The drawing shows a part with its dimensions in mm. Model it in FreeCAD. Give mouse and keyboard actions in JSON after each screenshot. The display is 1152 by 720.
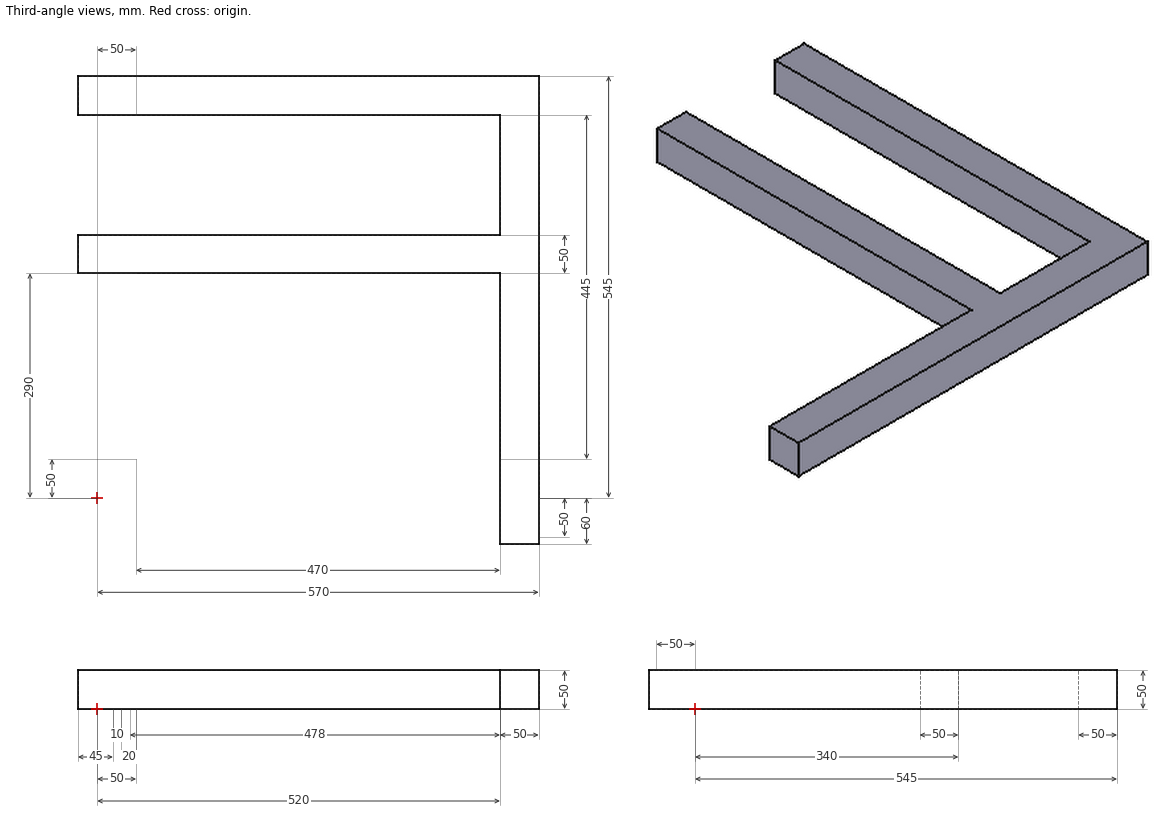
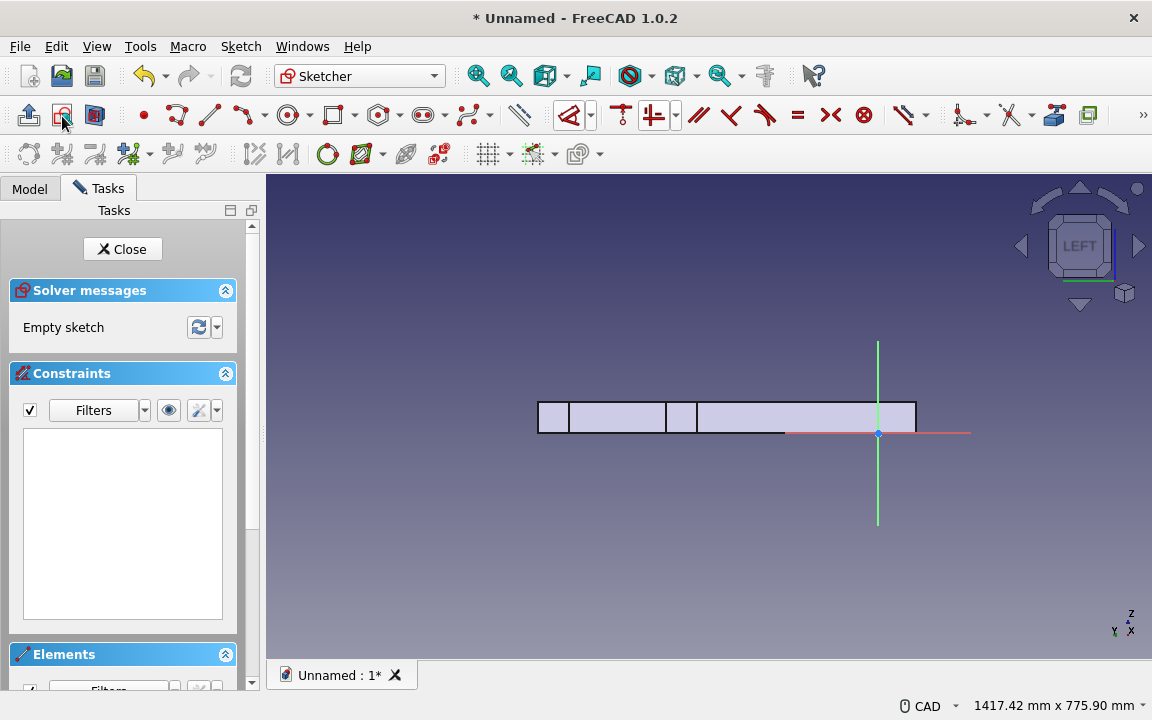
{"action": "scroll", "coordinate": [845, 420], "scroll_direction": "up", "scroll_amount": 2}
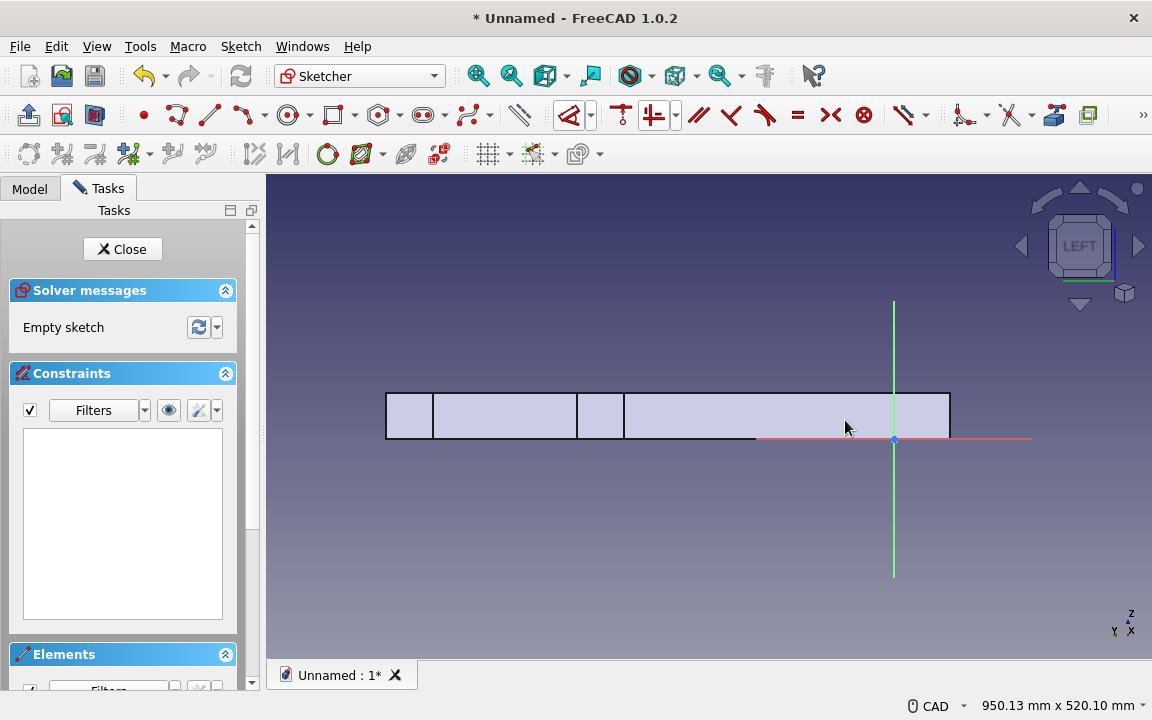
{"action": "key", "text": "g r"}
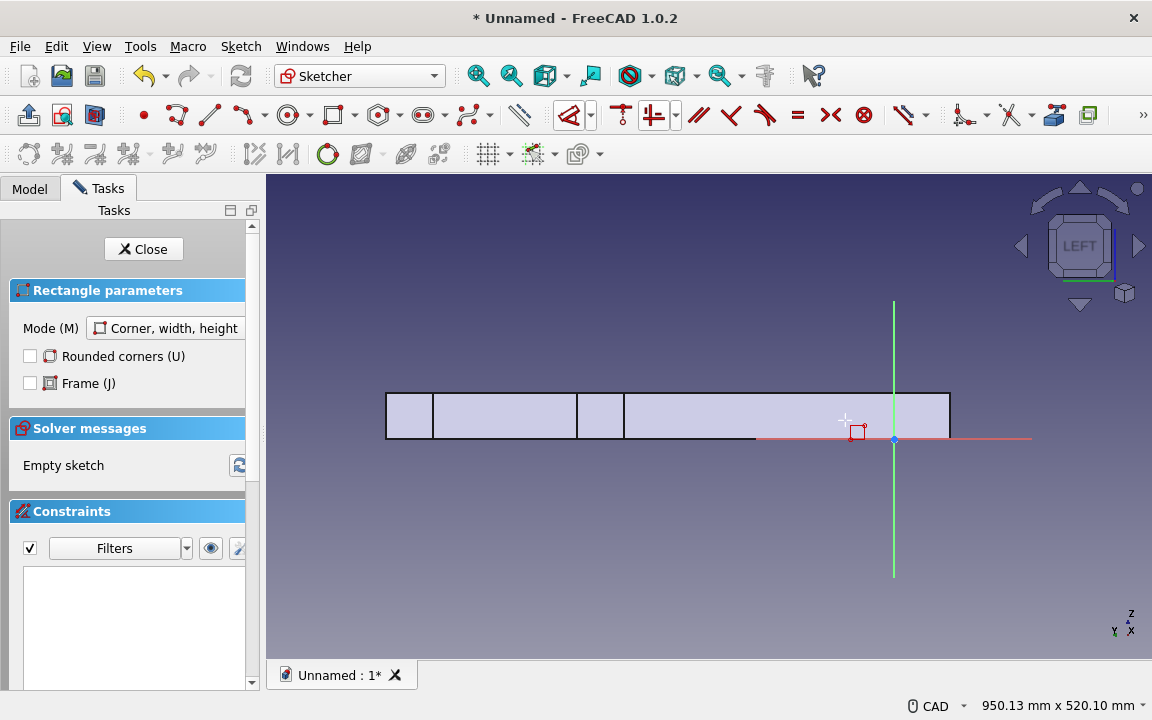
{"action": "left_click", "coordinate": [386, 393]}
{"action": "left_click", "coordinate": [433, 439]}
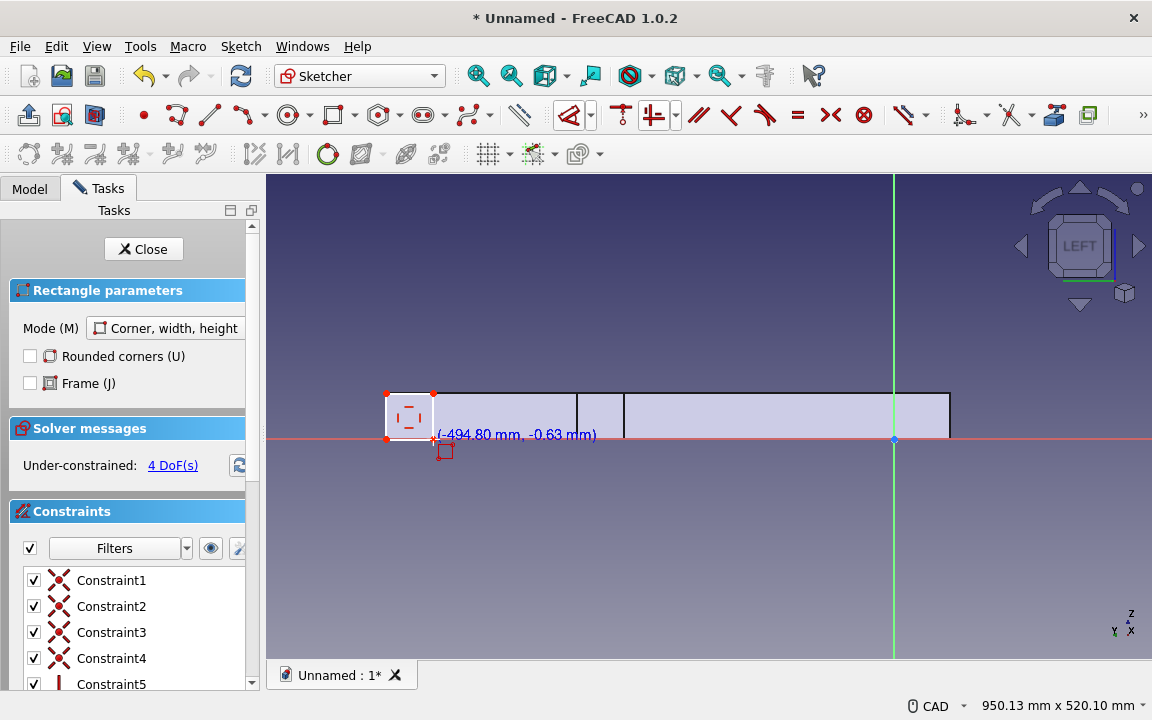
{"action": "left_click", "coordinate": [577, 393]}
{"action": "left_click", "coordinate": [624, 439]}
{"action": "key", "text": "Escape"}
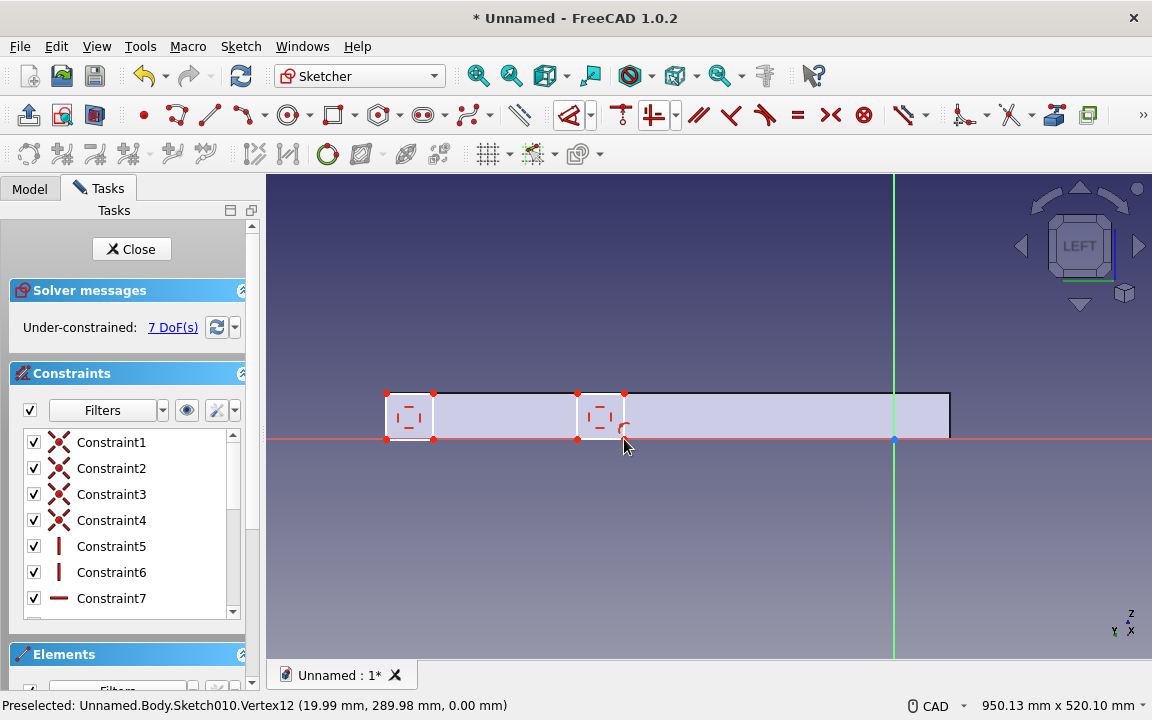
{"action": "left_click", "coordinate": [386, 440]}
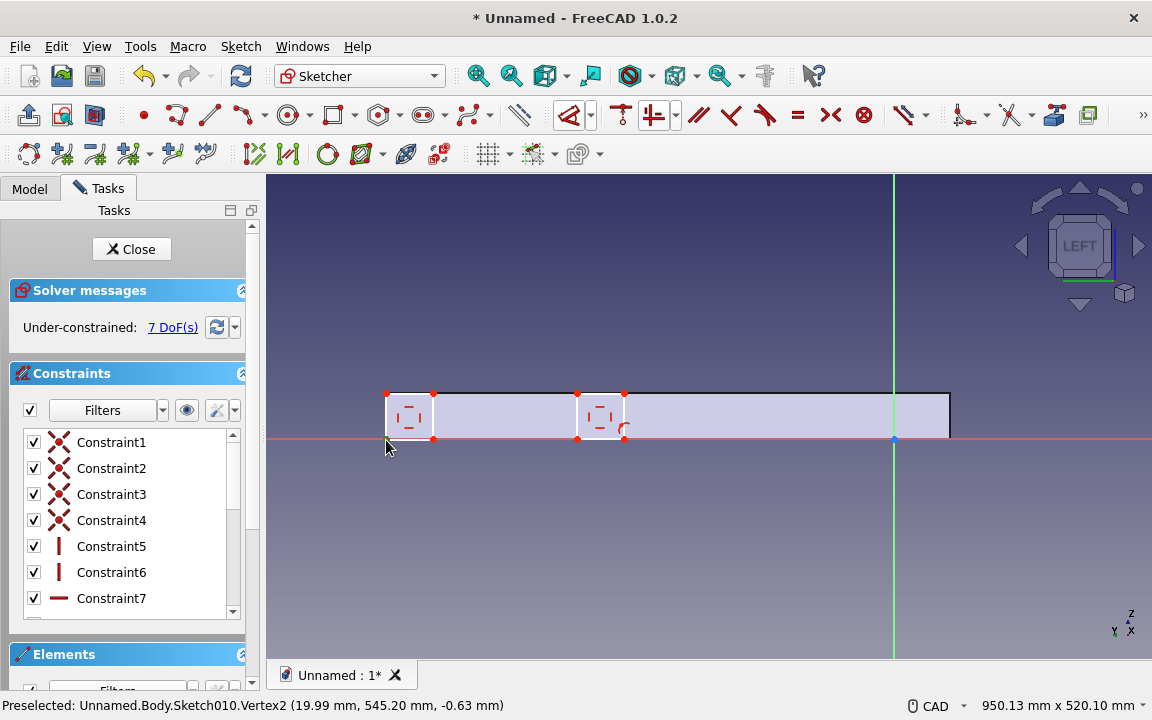
{"action": "left_click", "coordinate": [344, 439]}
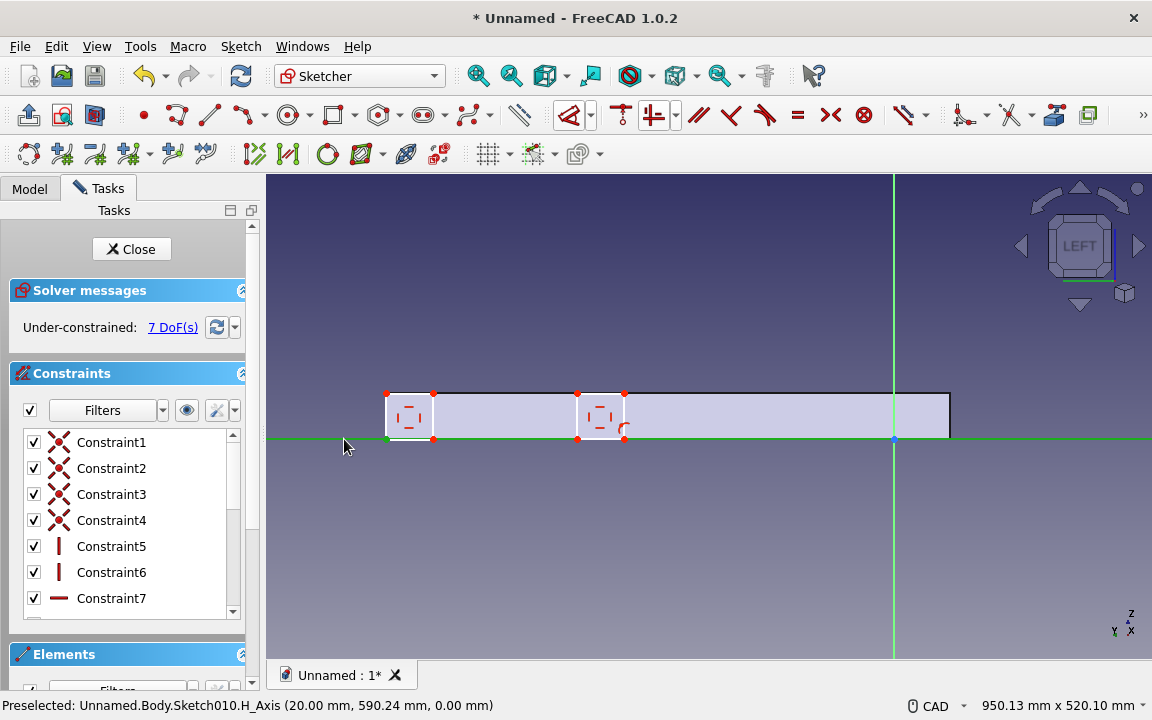
{"action": "left_click", "coordinate": [621, 116]}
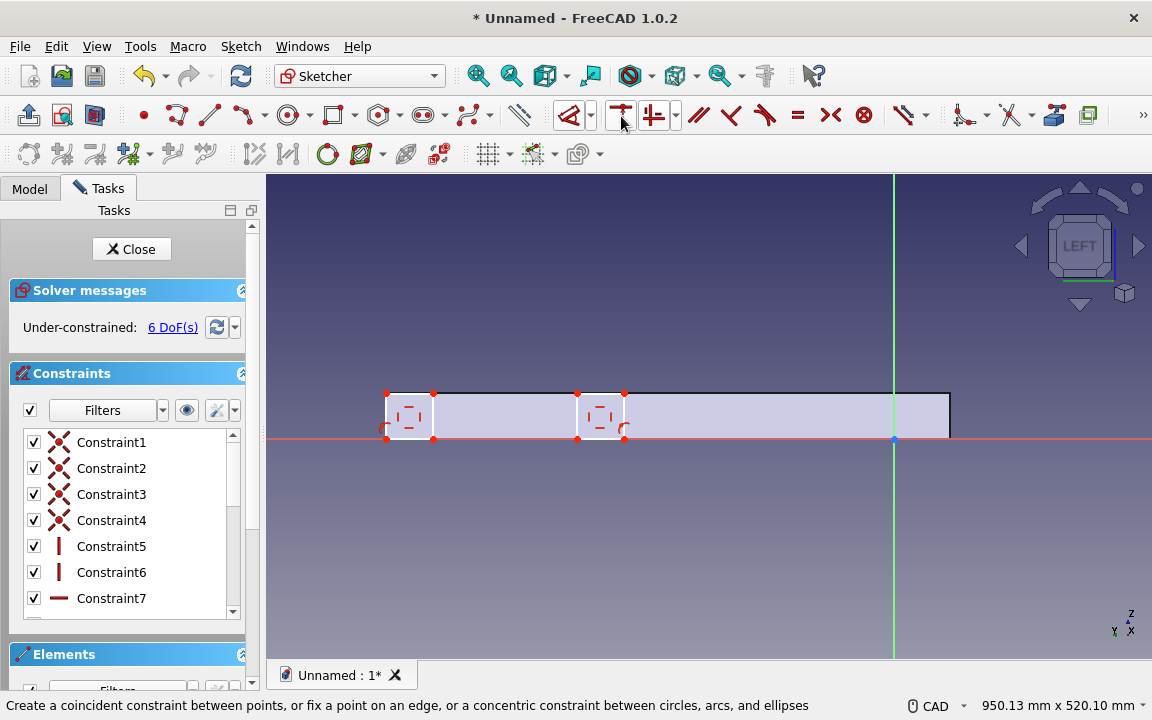
{"action": "left_click", "coordinate": [386, 408]}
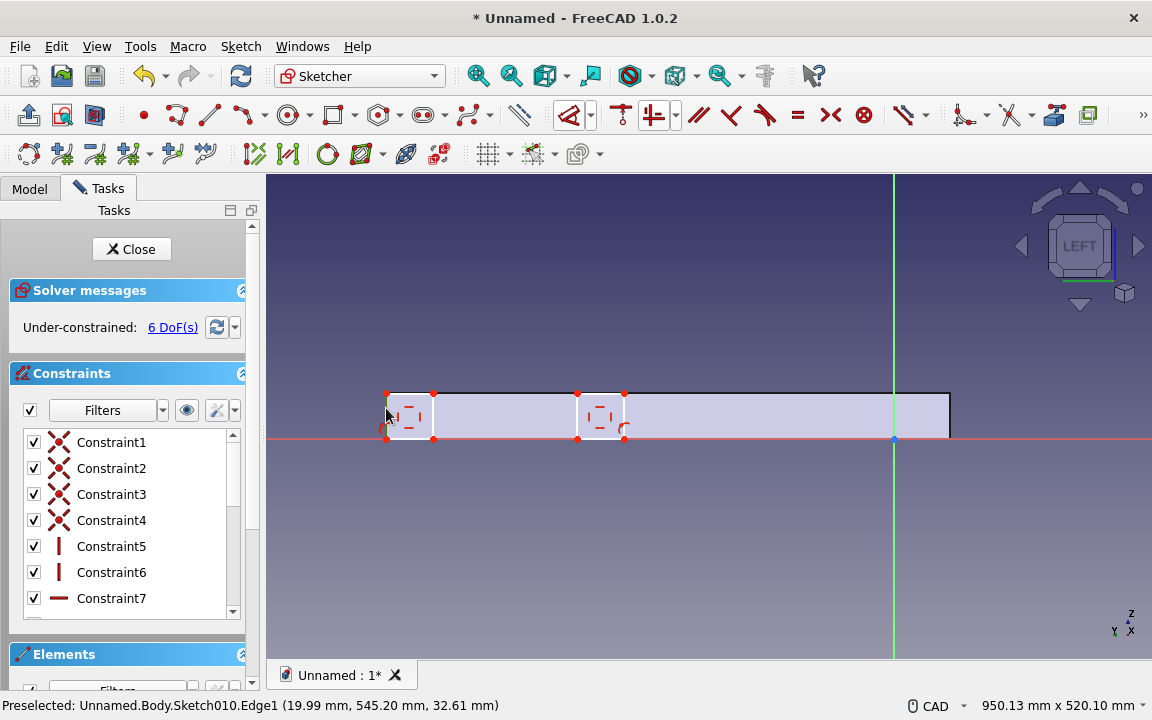
{"action": "key", "text": "i"}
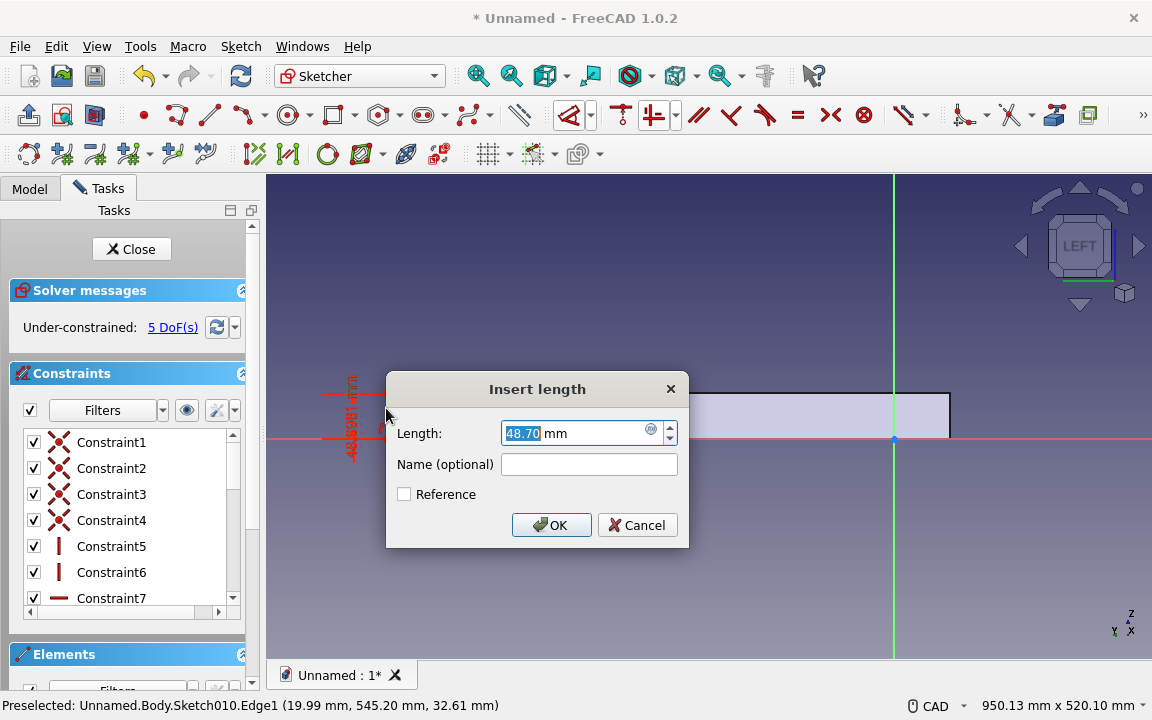
{"action": "type", "text": "50"}
{"action": "key", "text": "Return"}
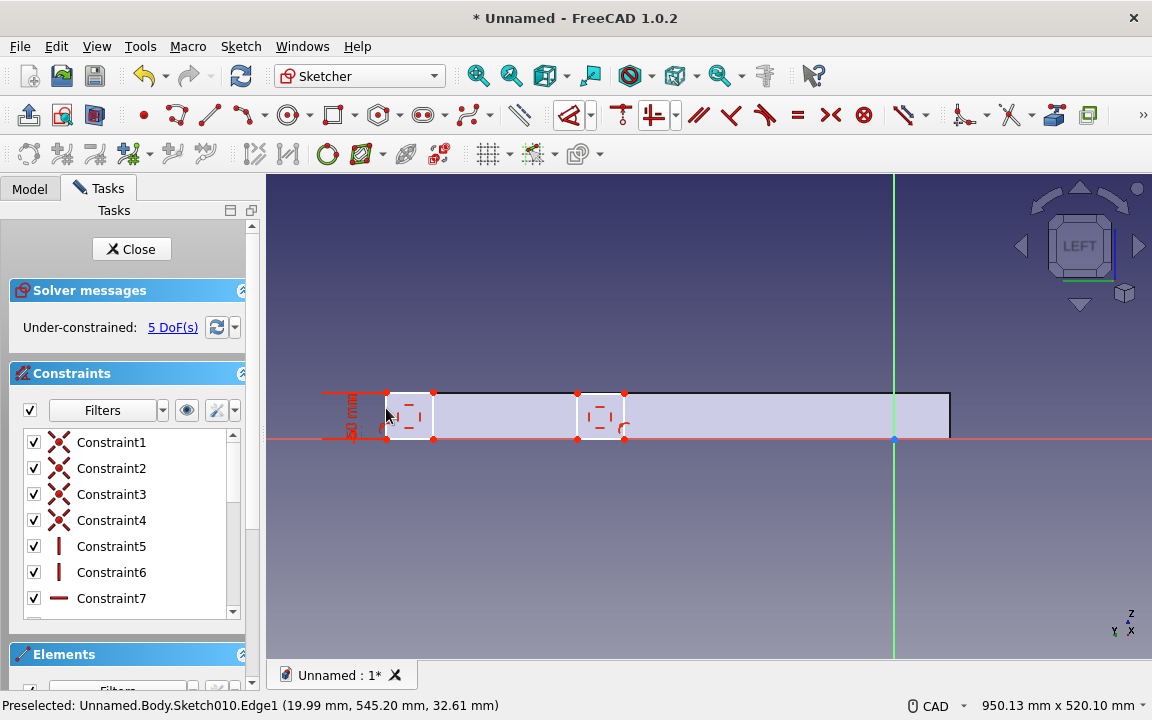
{"action": "left_click", "coordinate": [400, 439]}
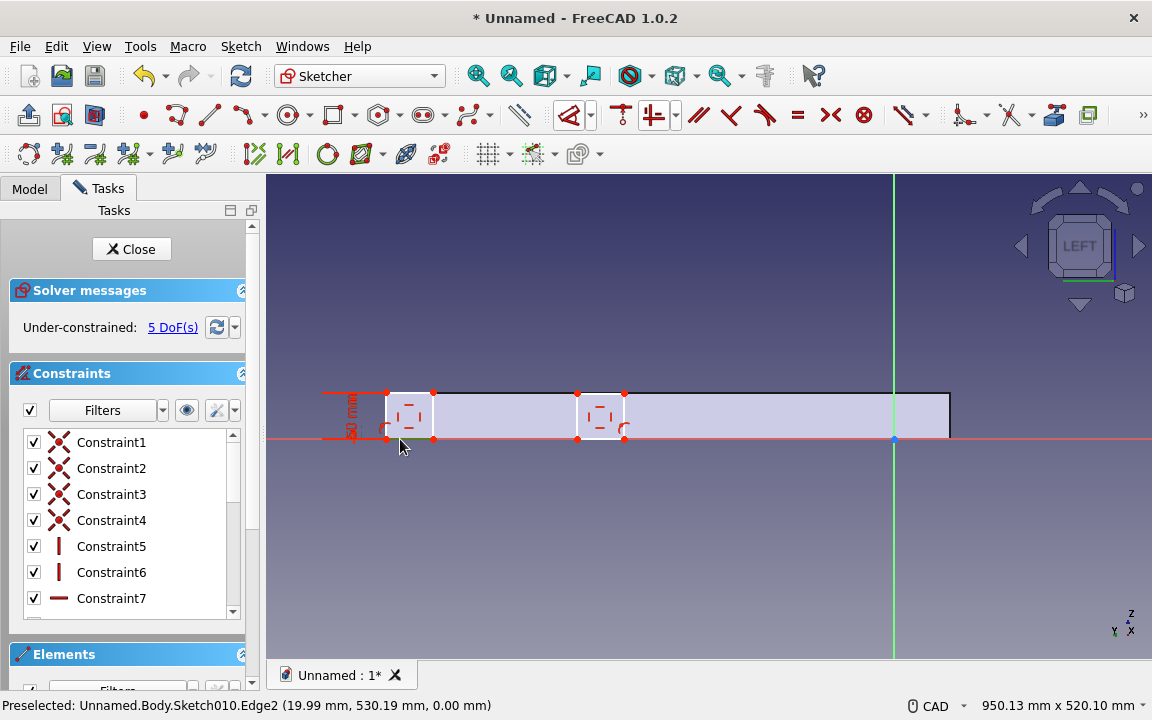
{"action": "key", "text": "l"}